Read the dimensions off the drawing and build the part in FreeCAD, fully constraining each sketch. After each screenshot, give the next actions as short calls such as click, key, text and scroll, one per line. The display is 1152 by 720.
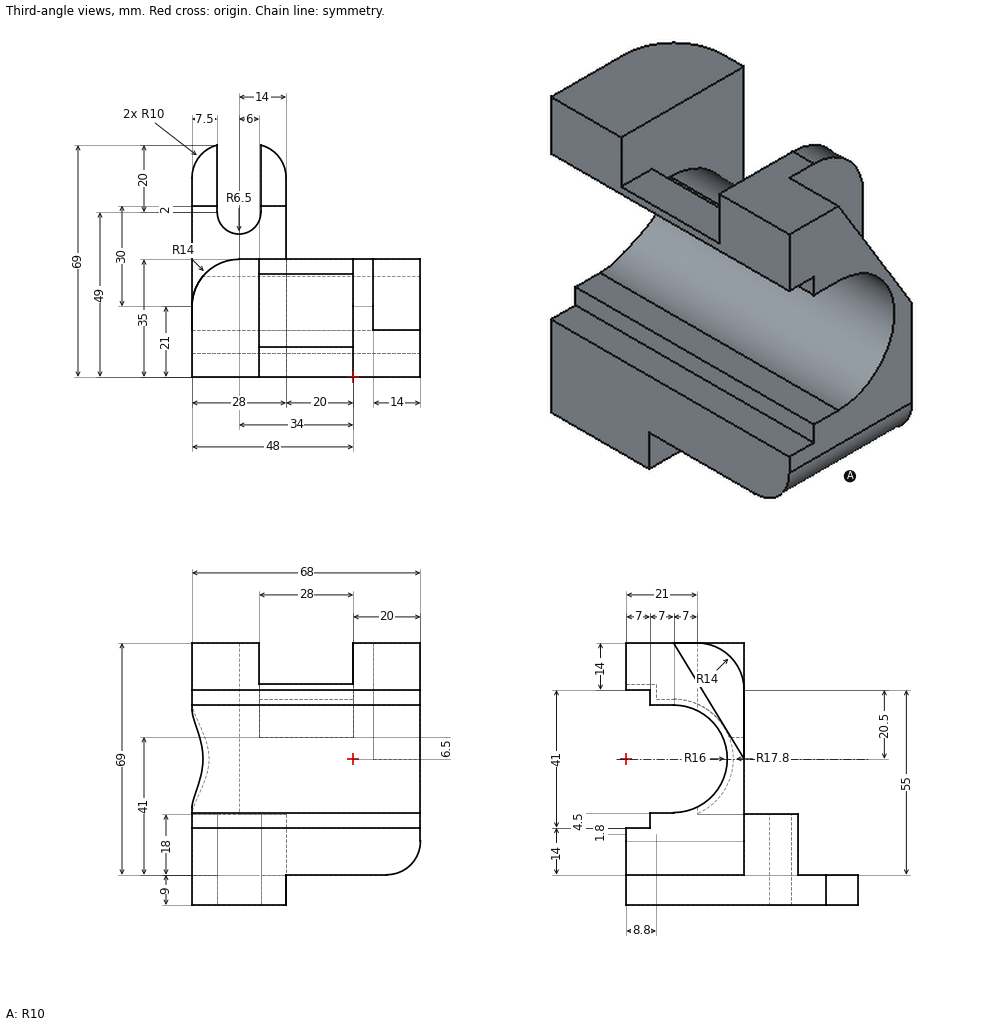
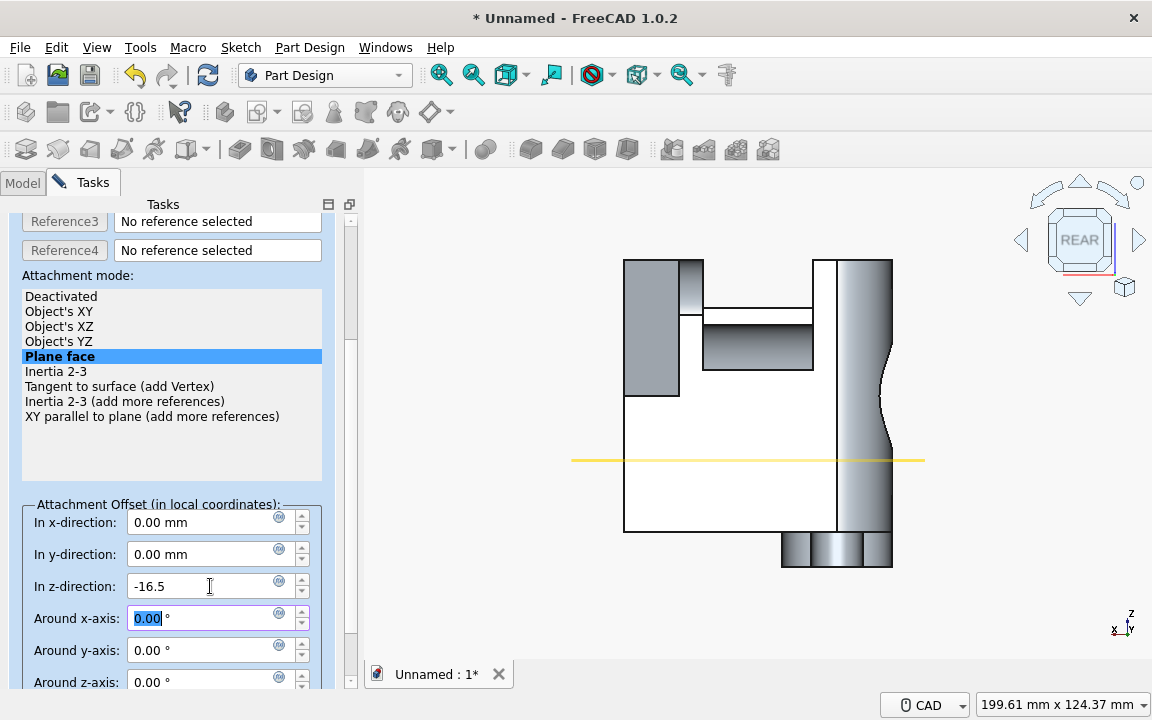
scroll(351, 451, up, 4)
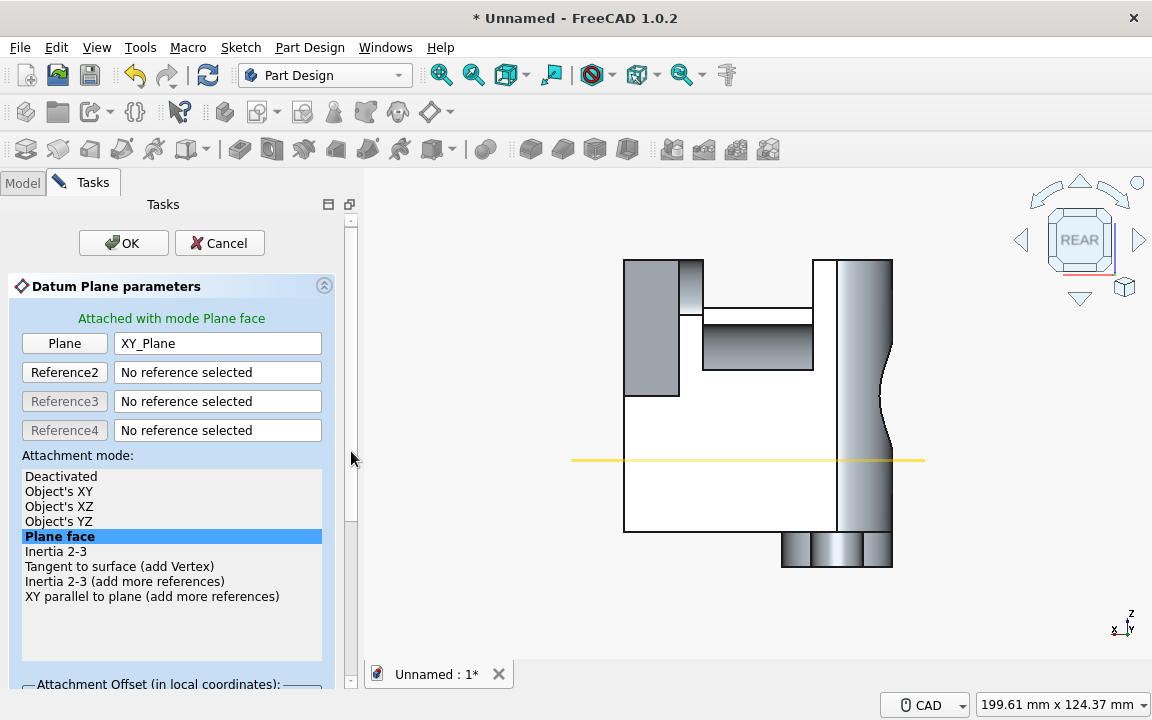
click(124, 243)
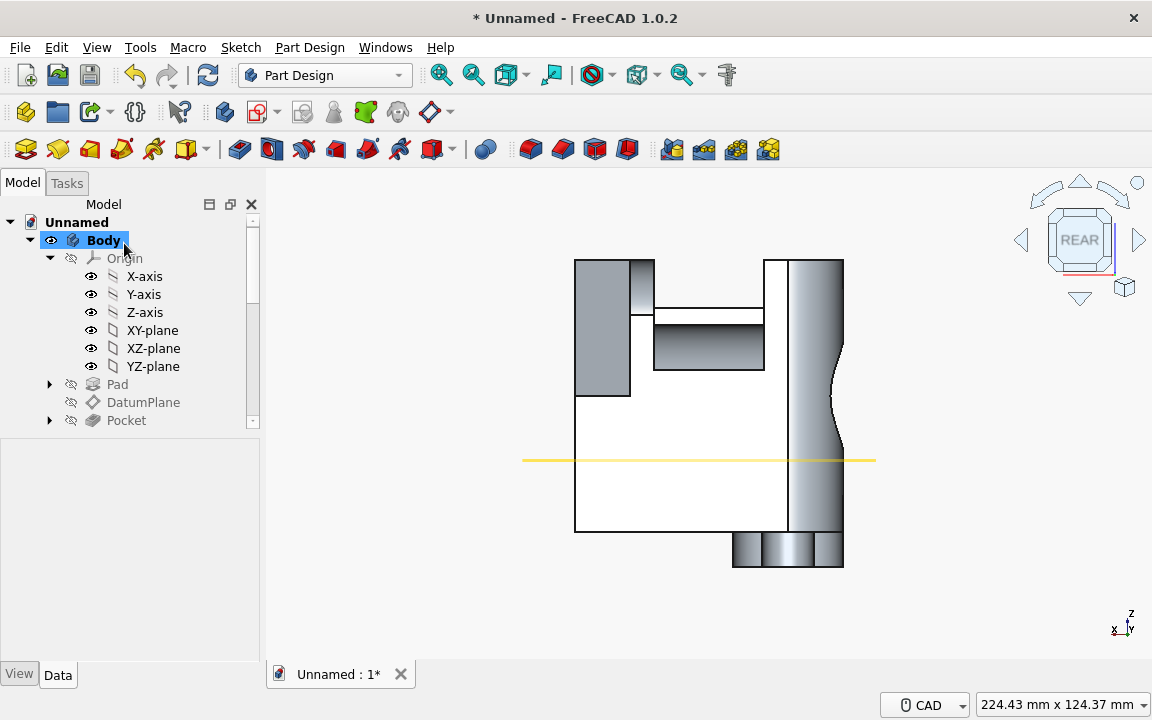
scroll(100, 326, down, 3)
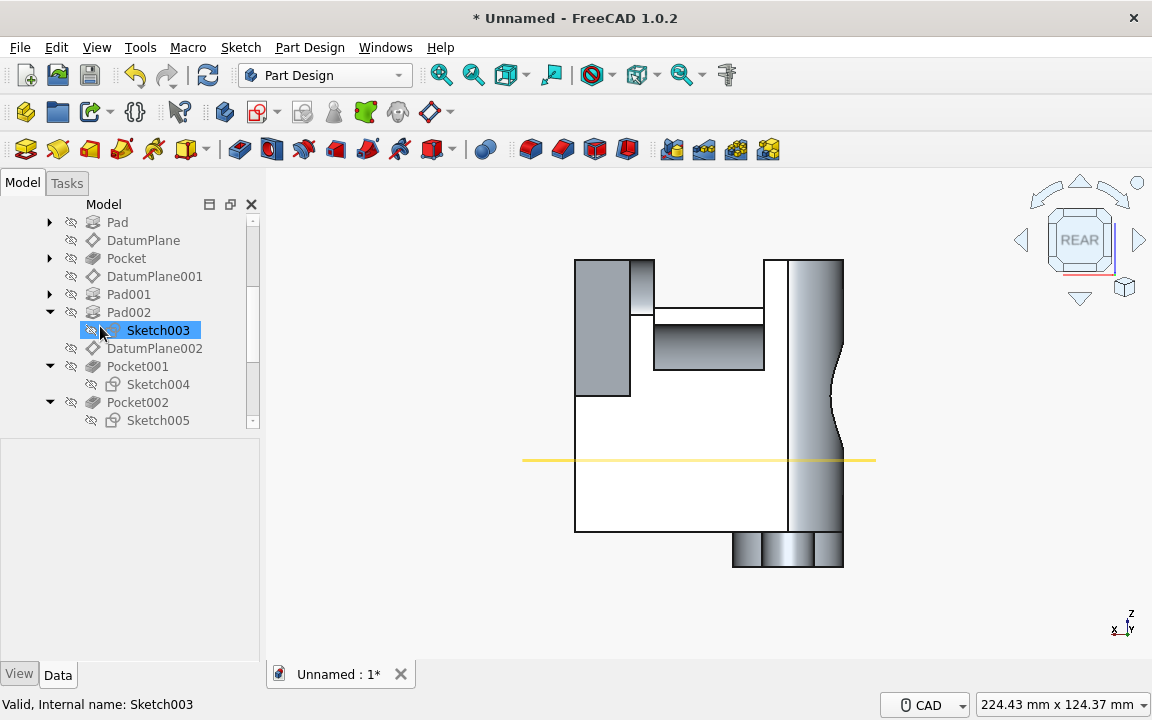
scroll(140, 326, up, 15)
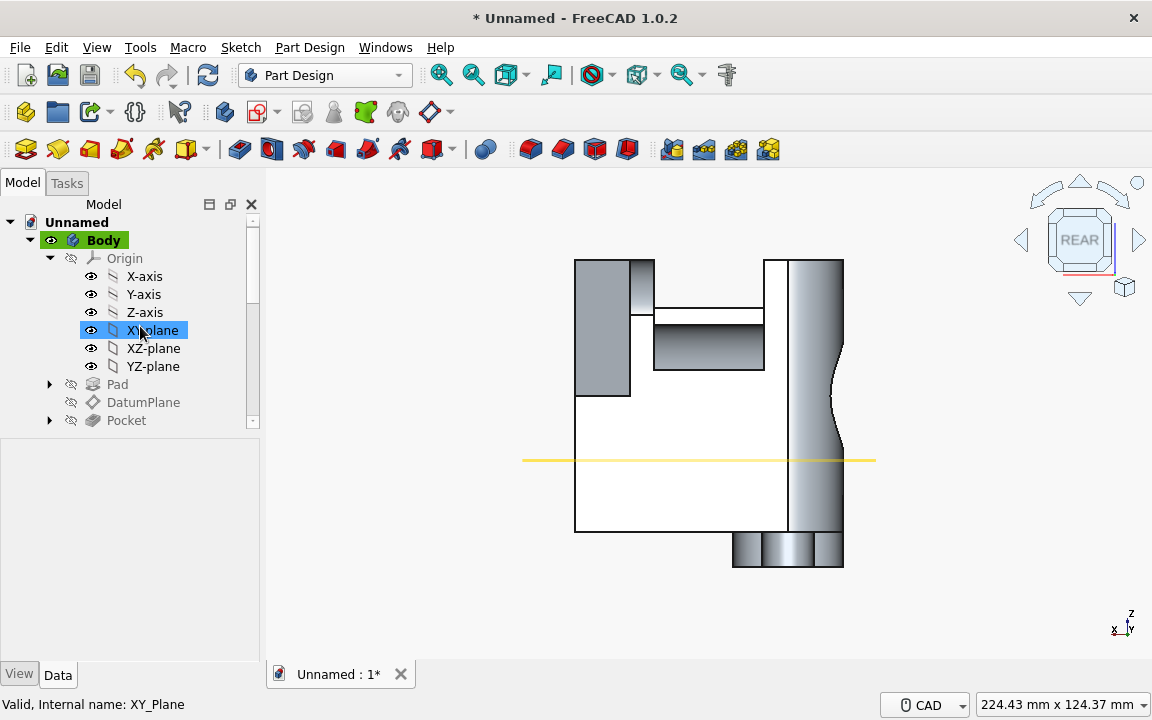
scroll(100, 326, down, 6)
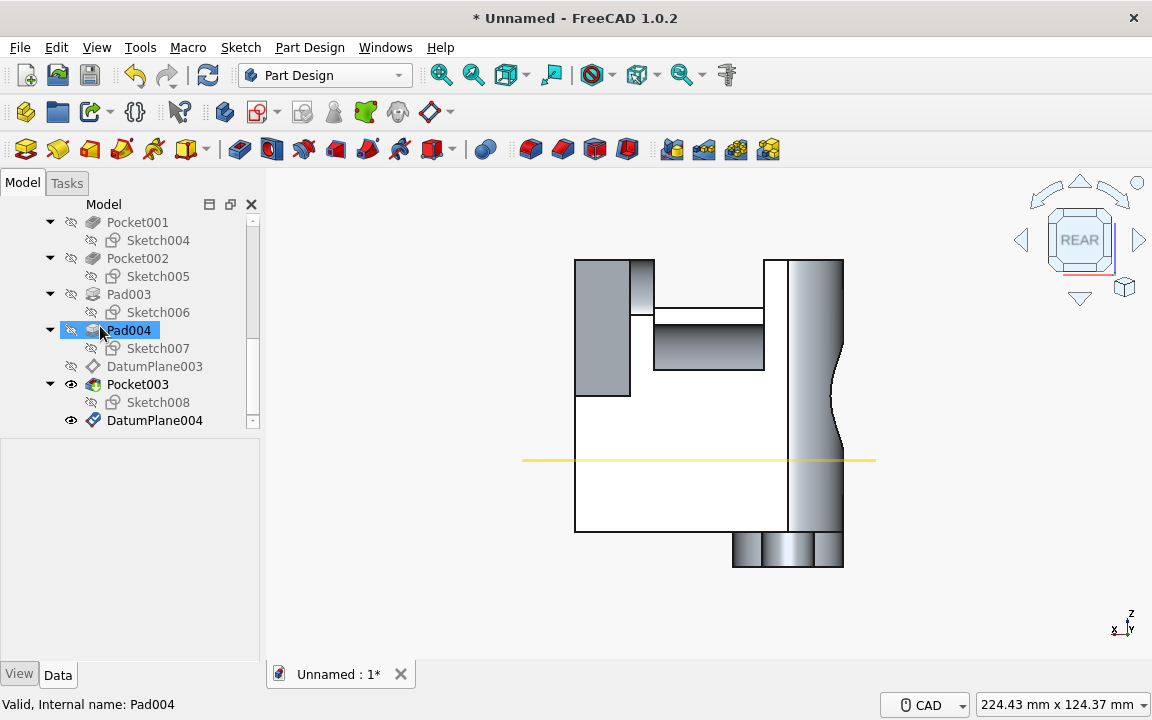
click(116, 420)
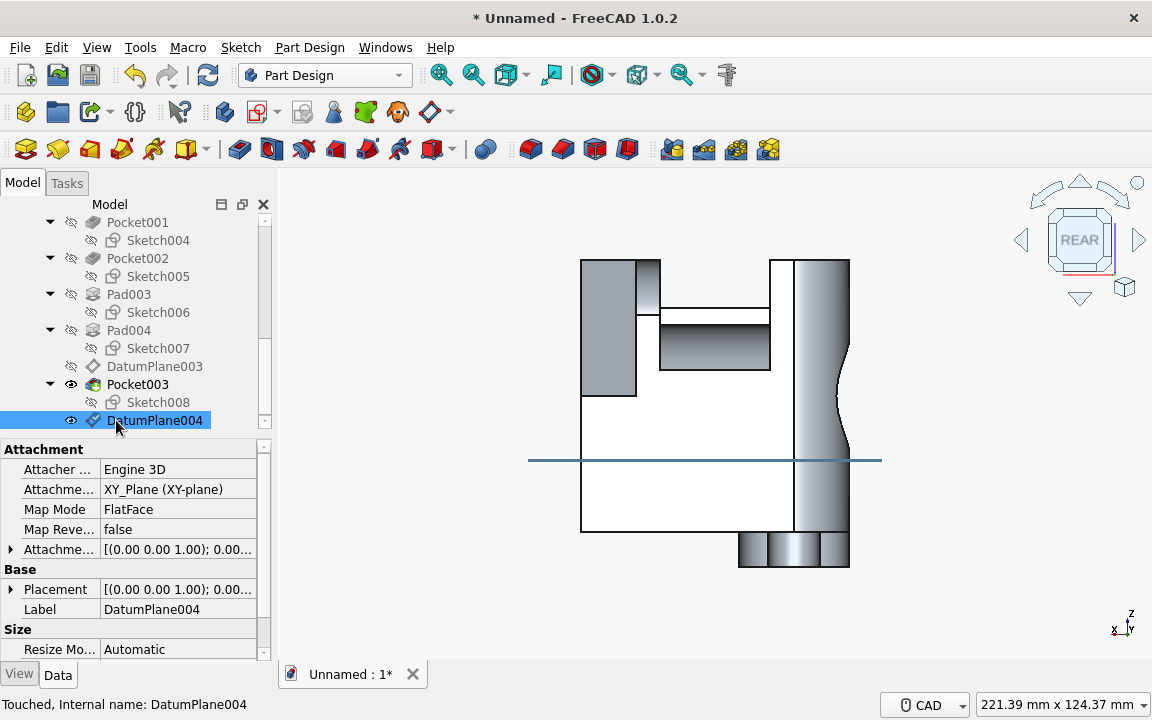
click(258, 112)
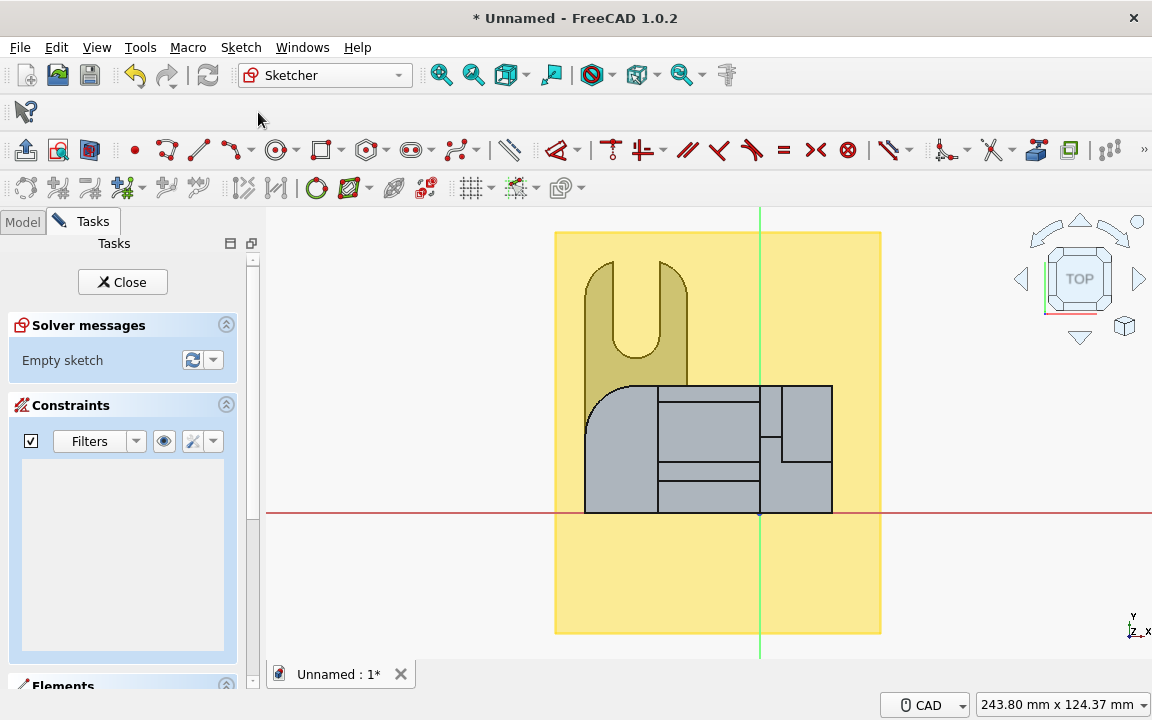
click(90, 150)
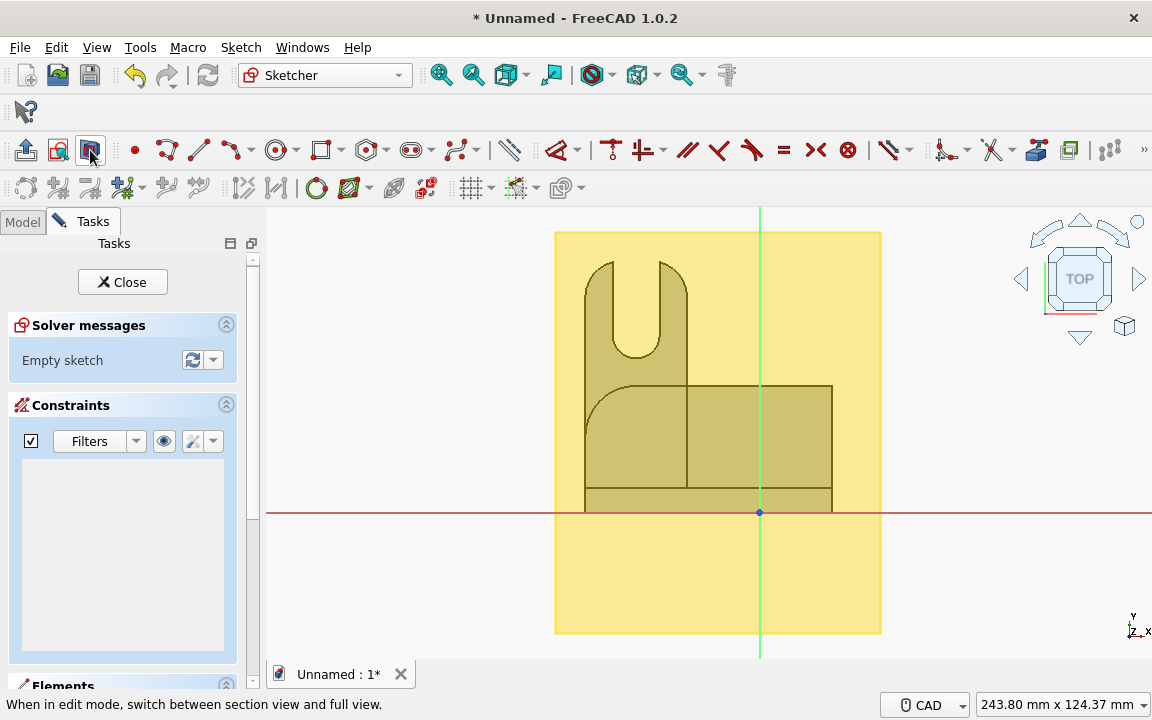
scroll(738, 394, up, 2)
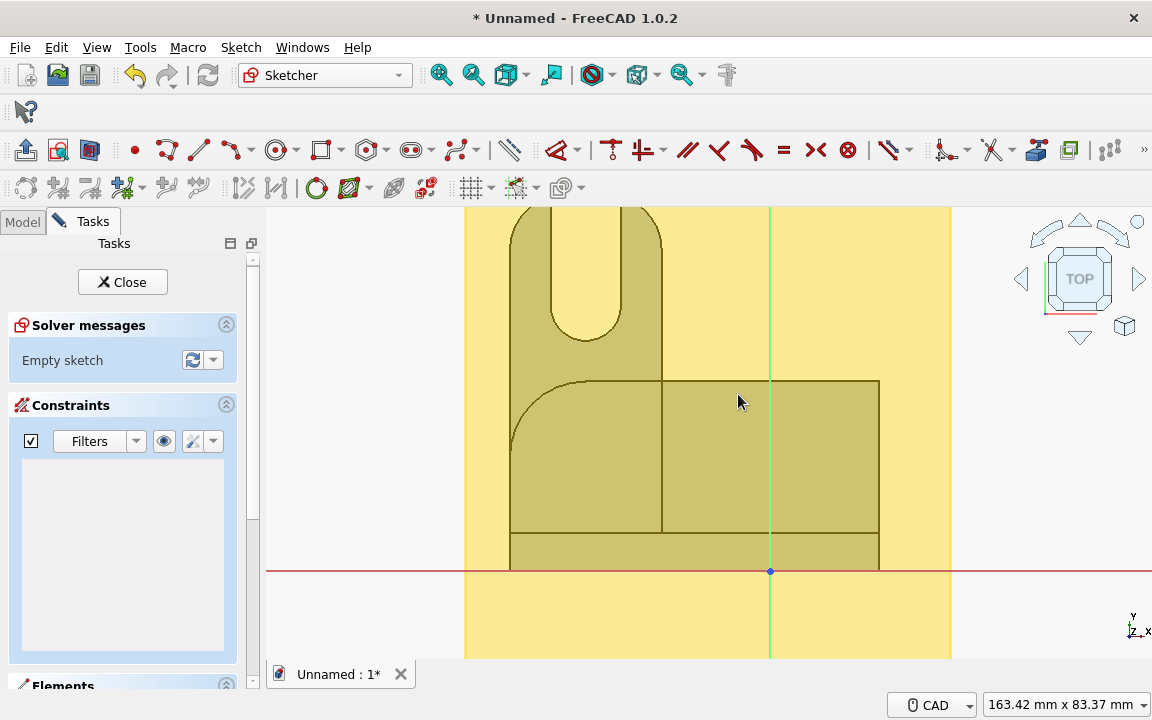
click(168, 150)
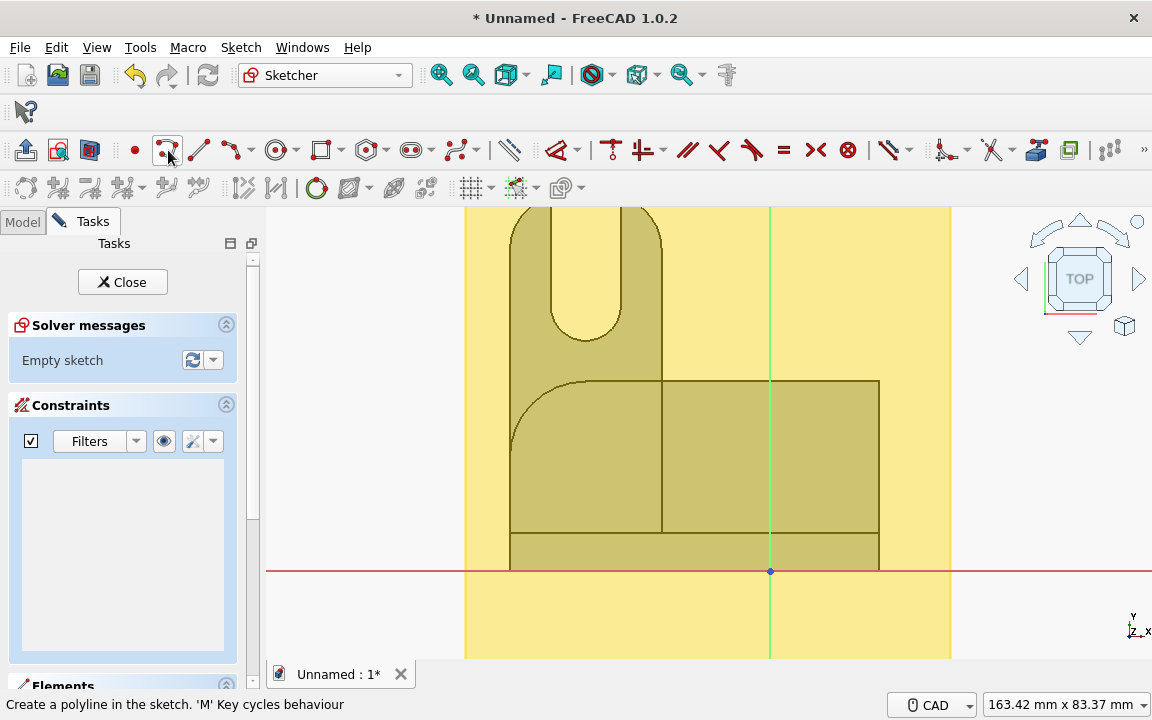
click(551, 306)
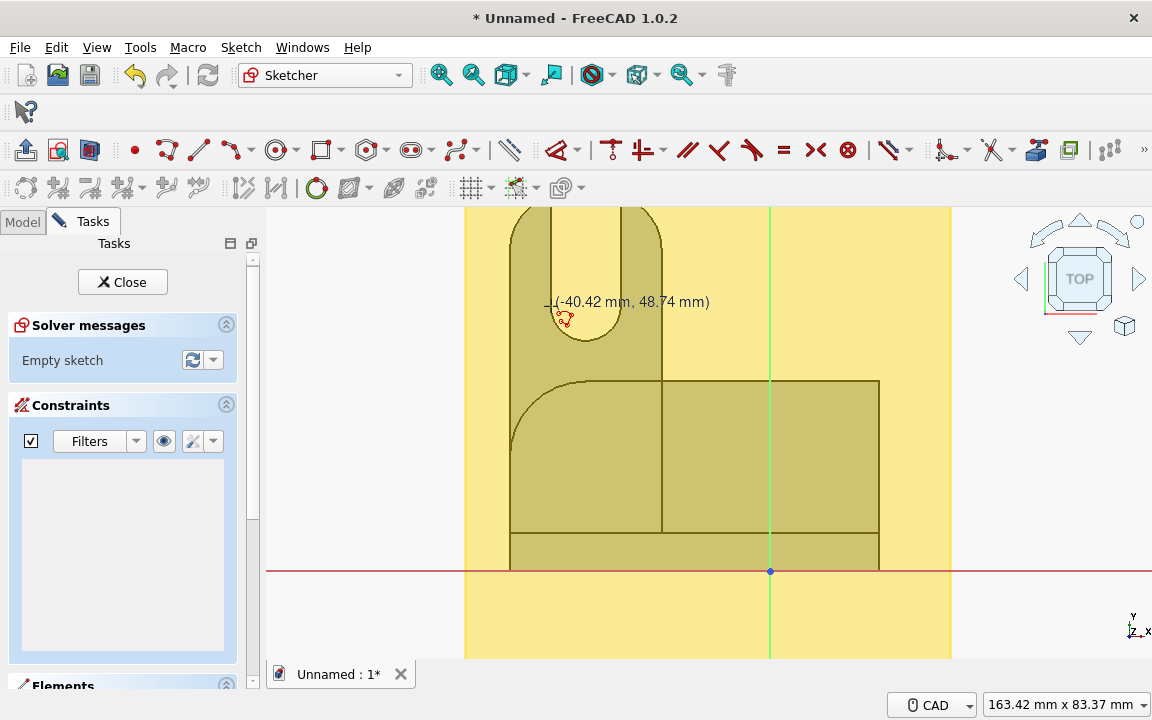
scroll(551, 295, up, 2)